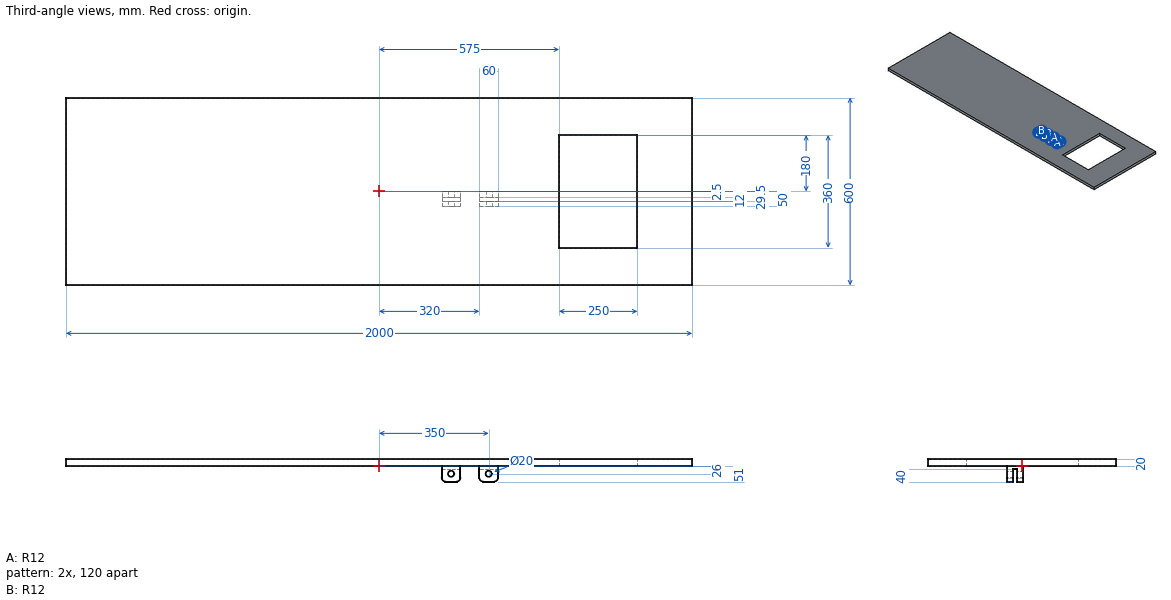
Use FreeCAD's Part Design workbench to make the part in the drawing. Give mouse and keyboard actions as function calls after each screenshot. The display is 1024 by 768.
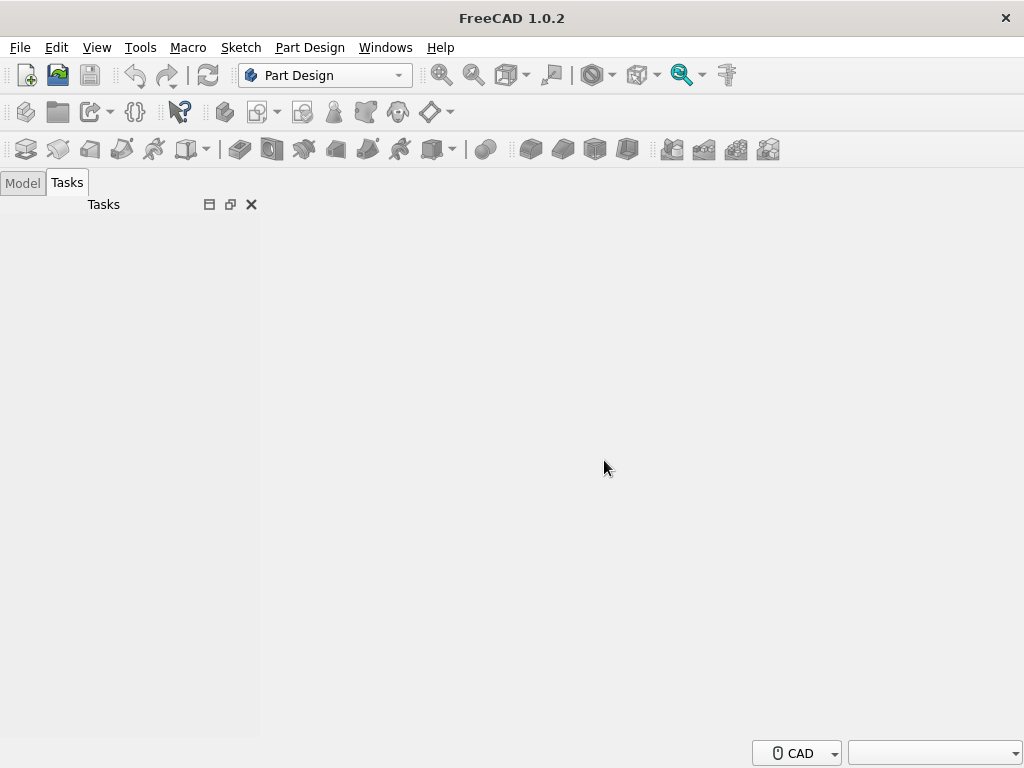
click(26, 76)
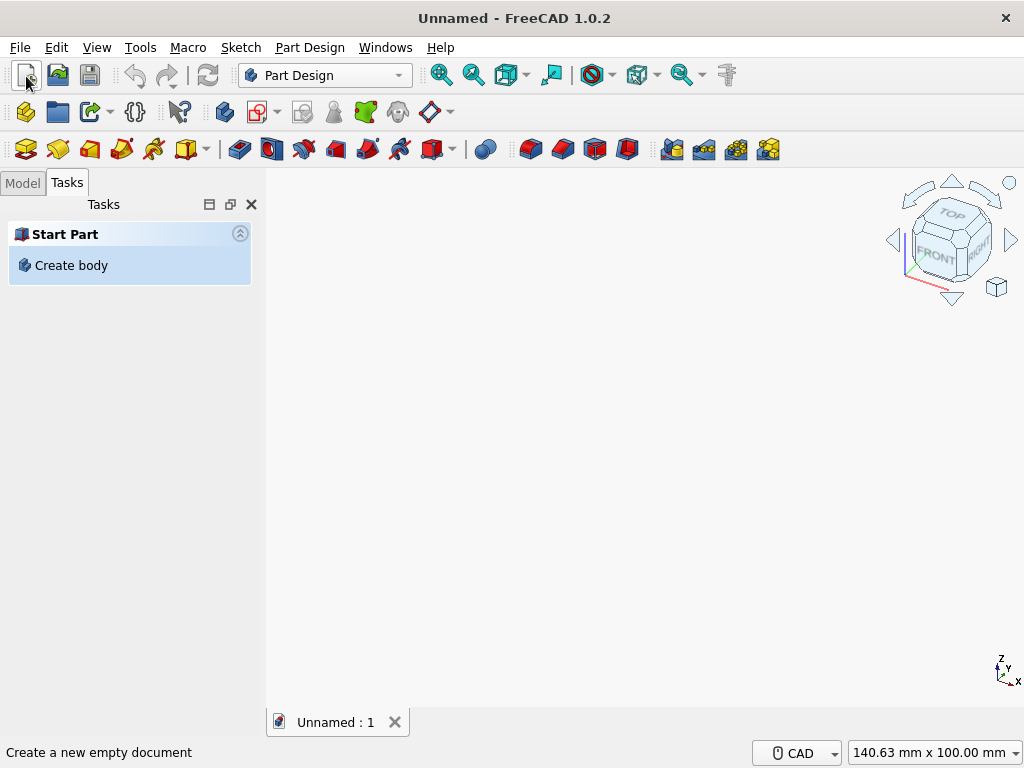
click(258, 112)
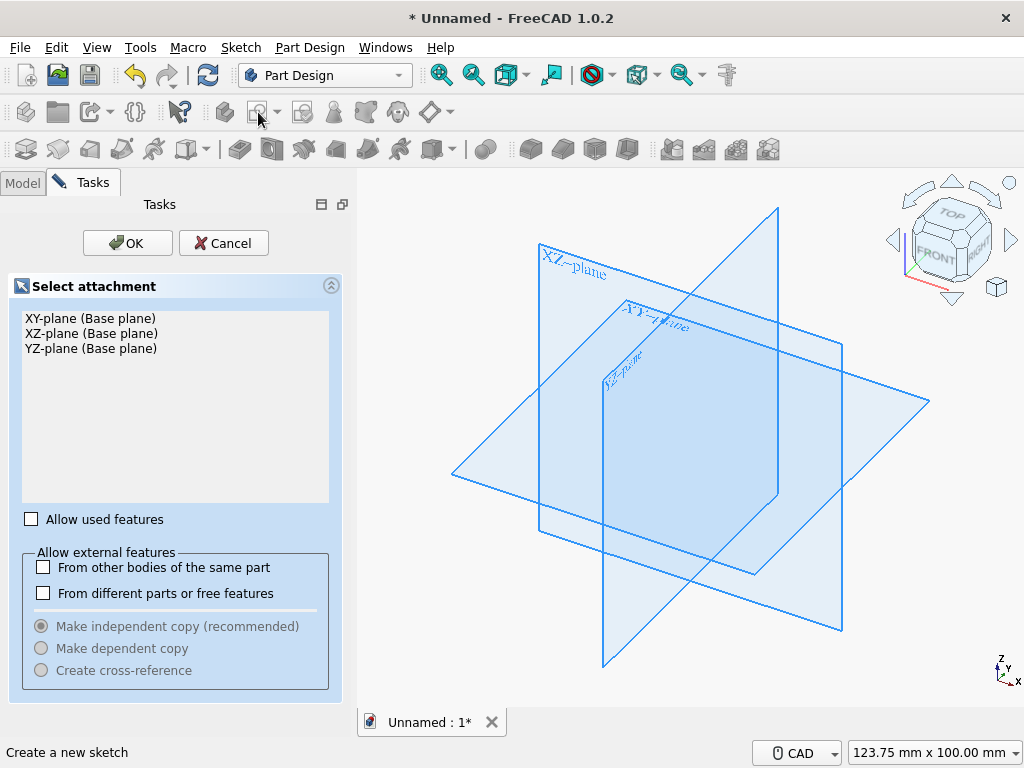
click(82, 318)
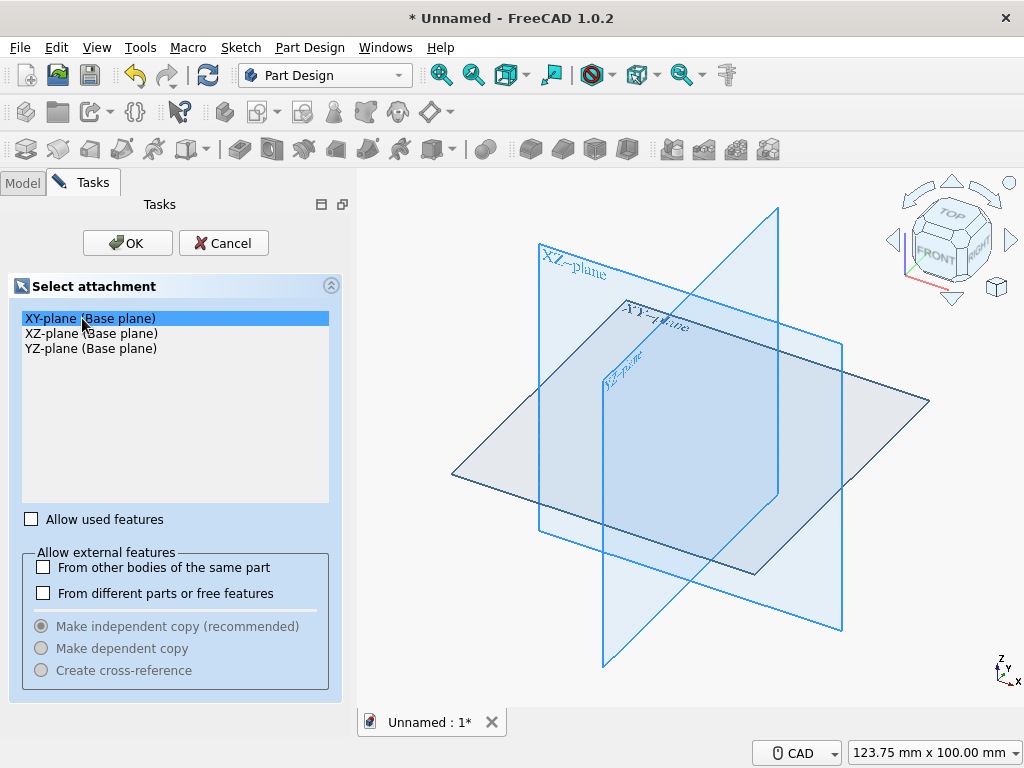
click(128, 243)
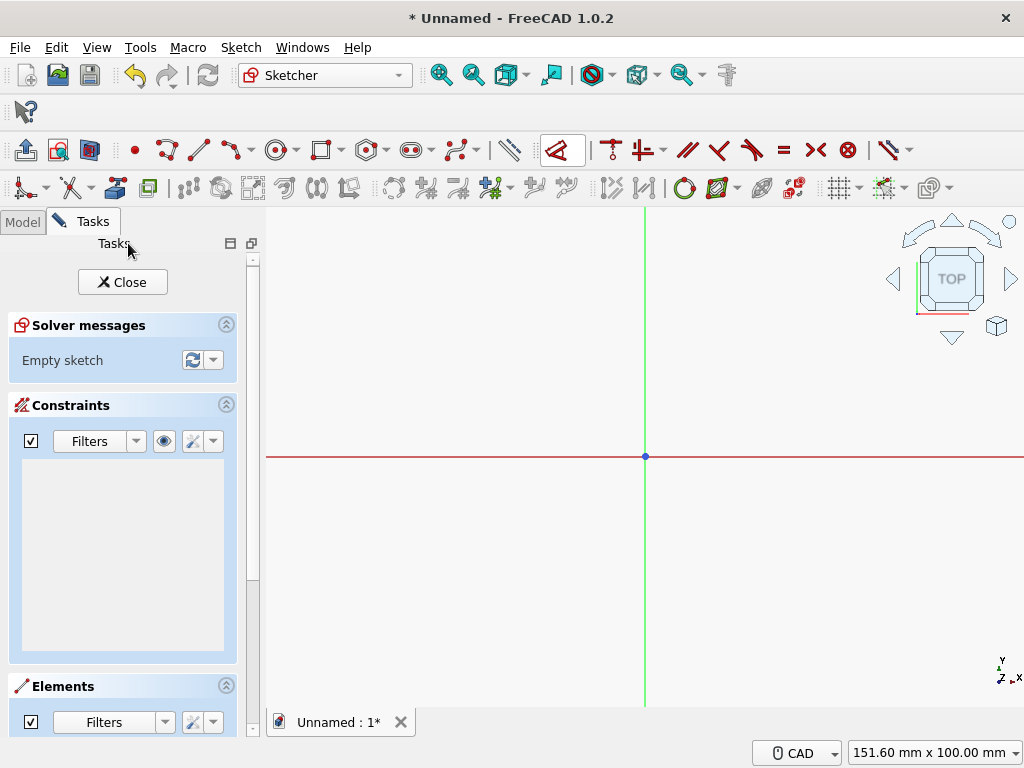
scroll(573, 457, down, 15)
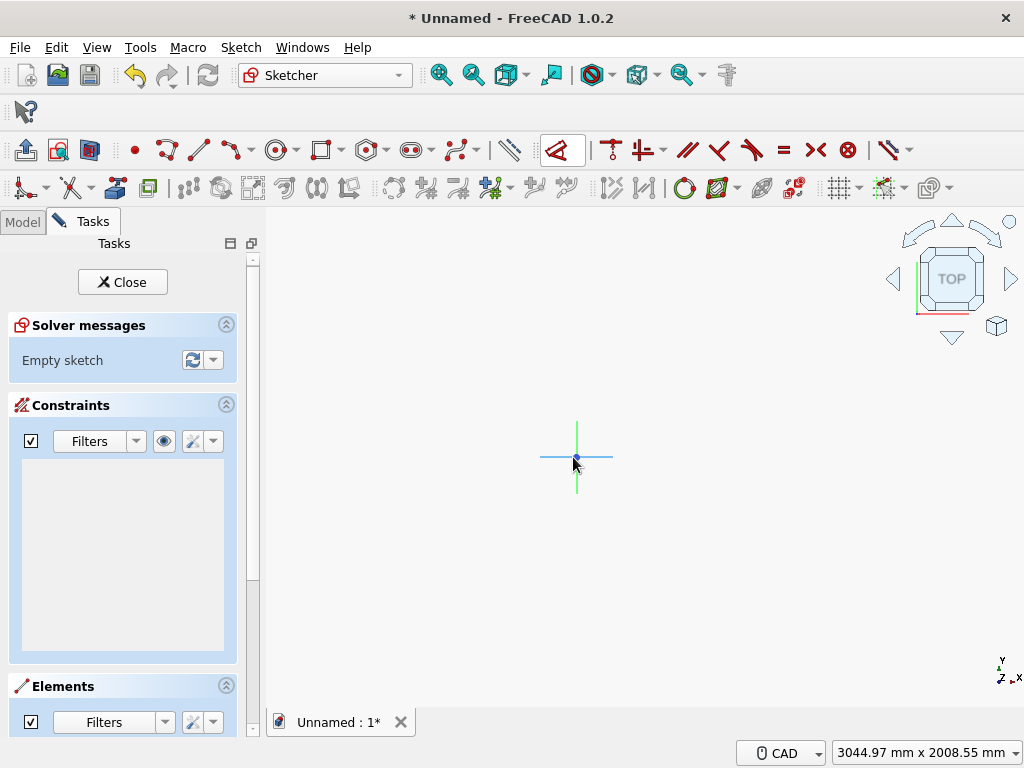
key(g)
key(v)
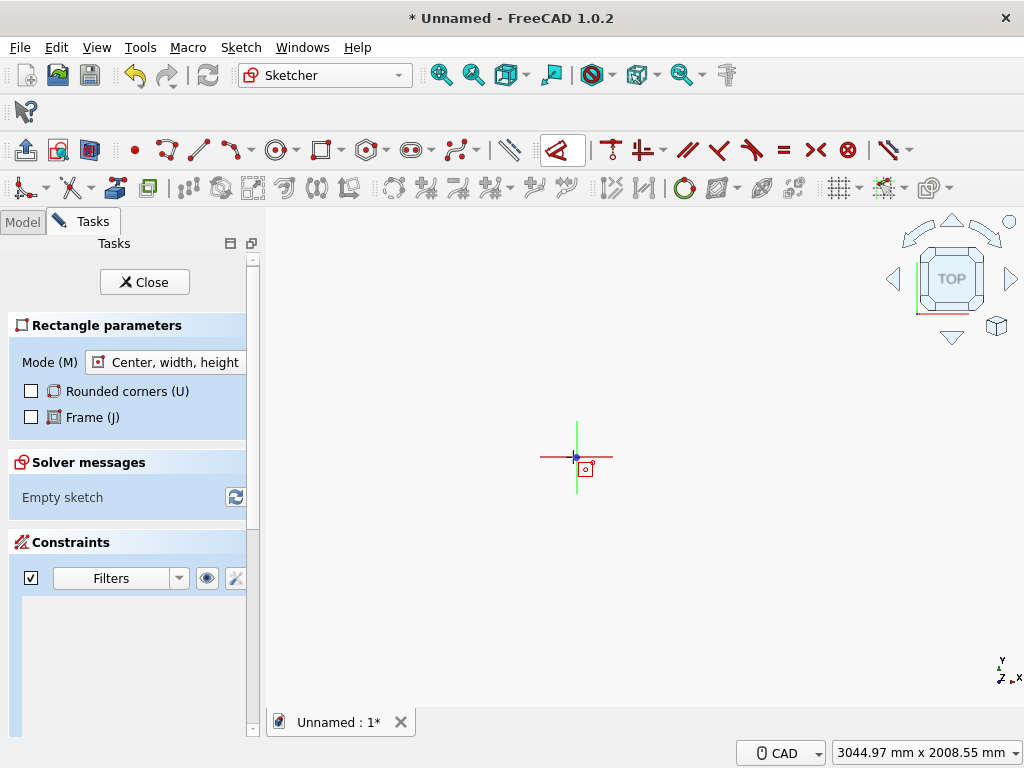
click(577, 457)
move(826, 383)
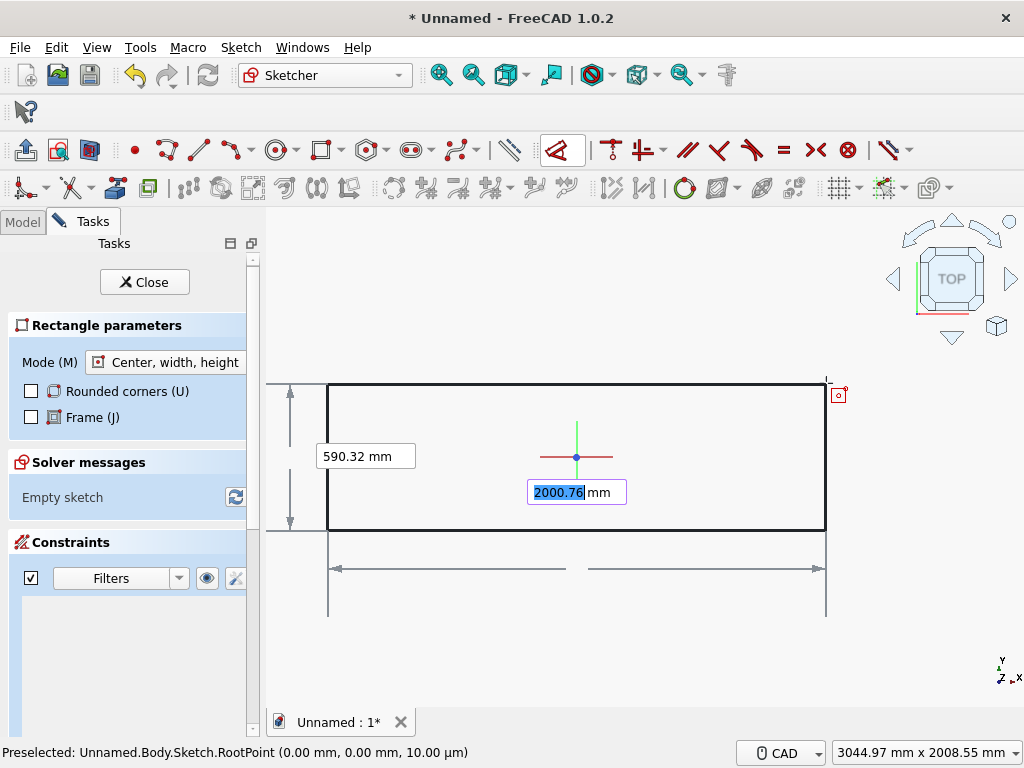
text(2000)
key(Tab)
text(600)
key(Return)
key(Escape)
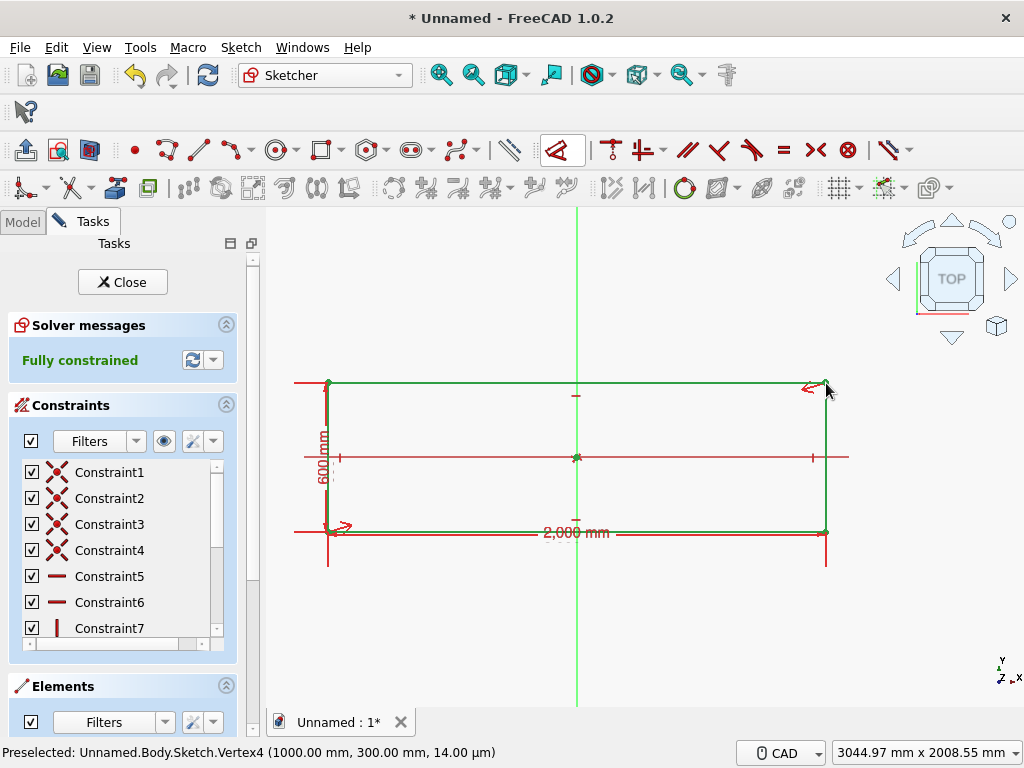
click(123, 282)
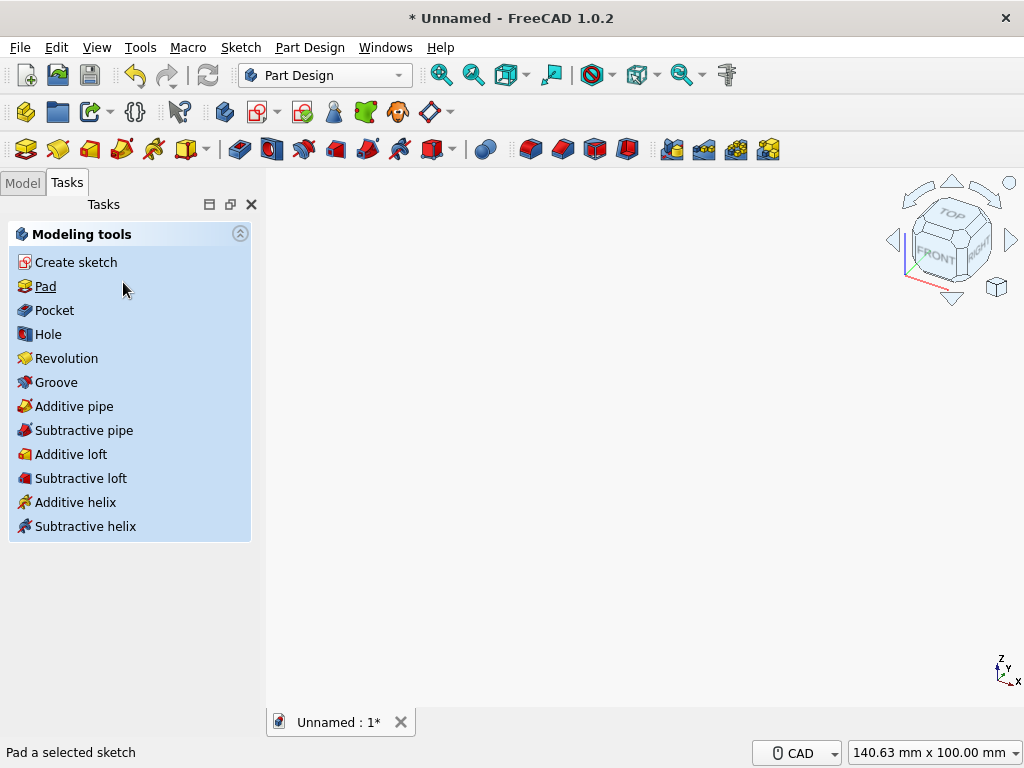
click(26, 150)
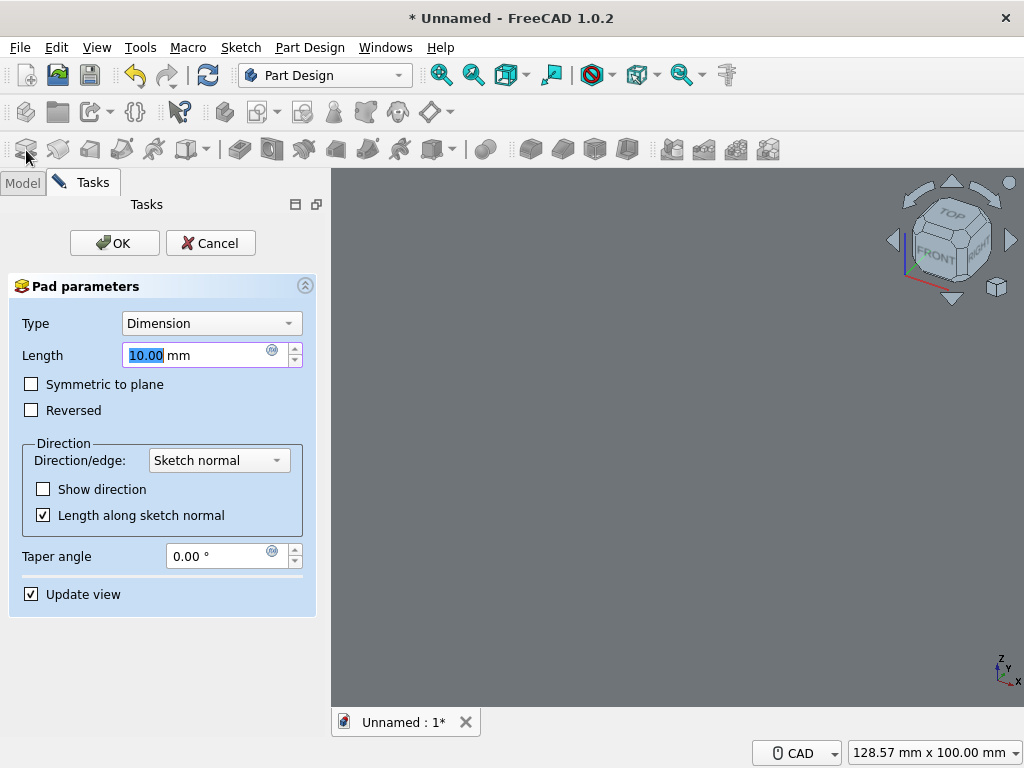
text(20)
key(Tab)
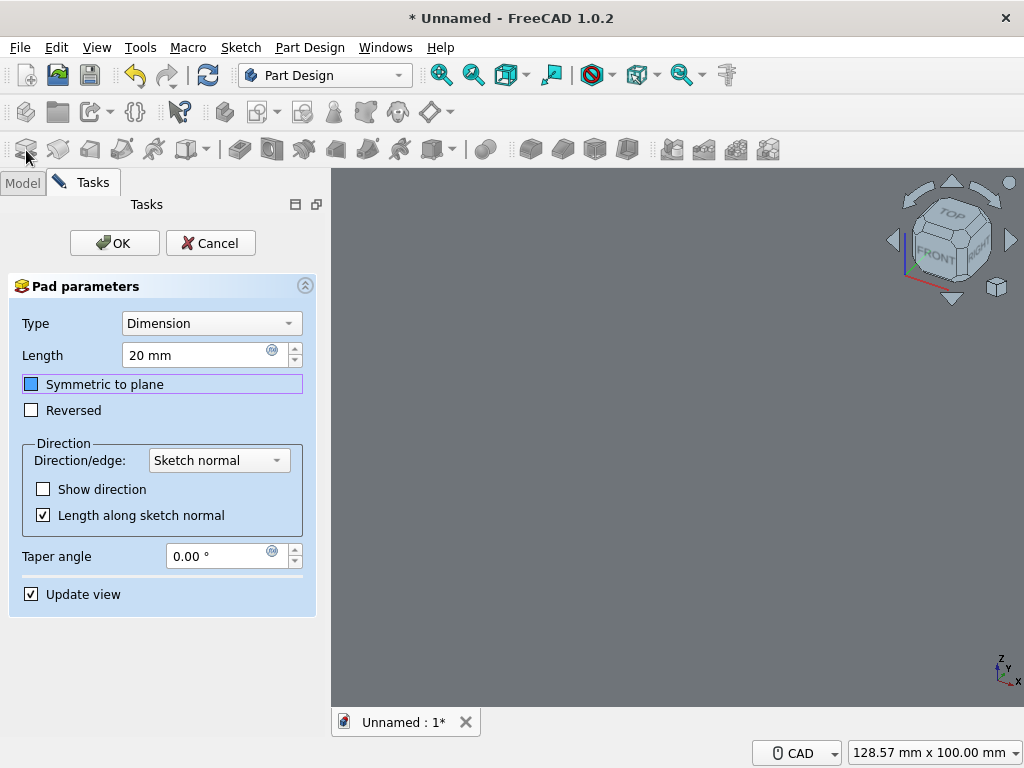
click(115, 243)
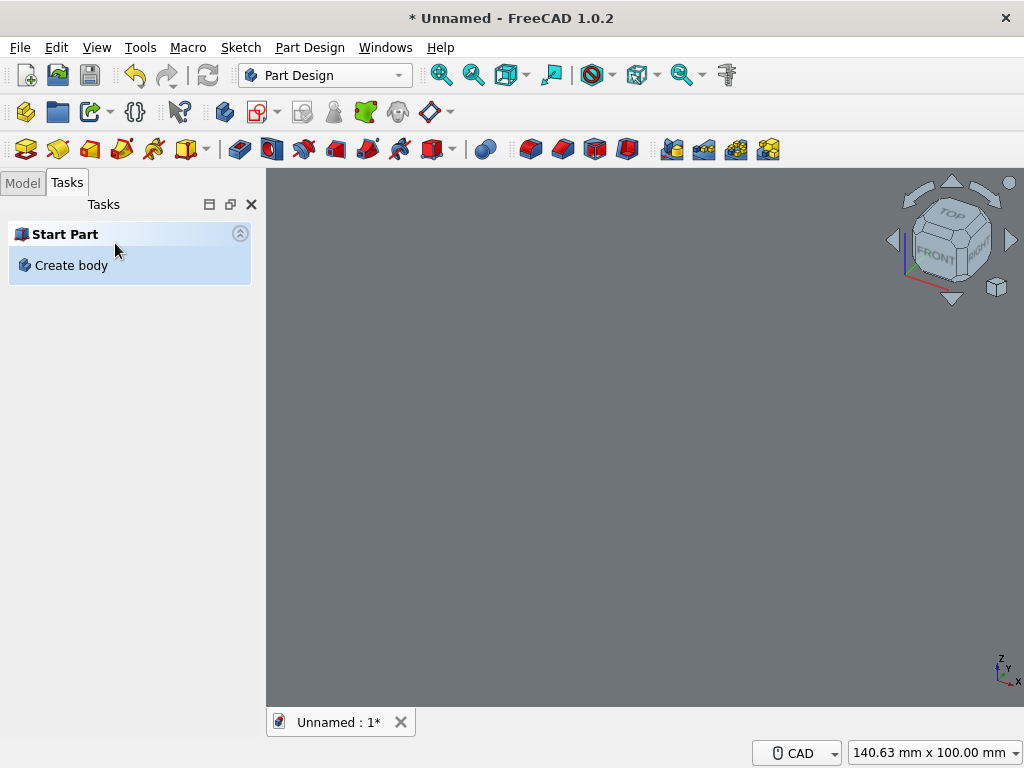
click(442, 76)